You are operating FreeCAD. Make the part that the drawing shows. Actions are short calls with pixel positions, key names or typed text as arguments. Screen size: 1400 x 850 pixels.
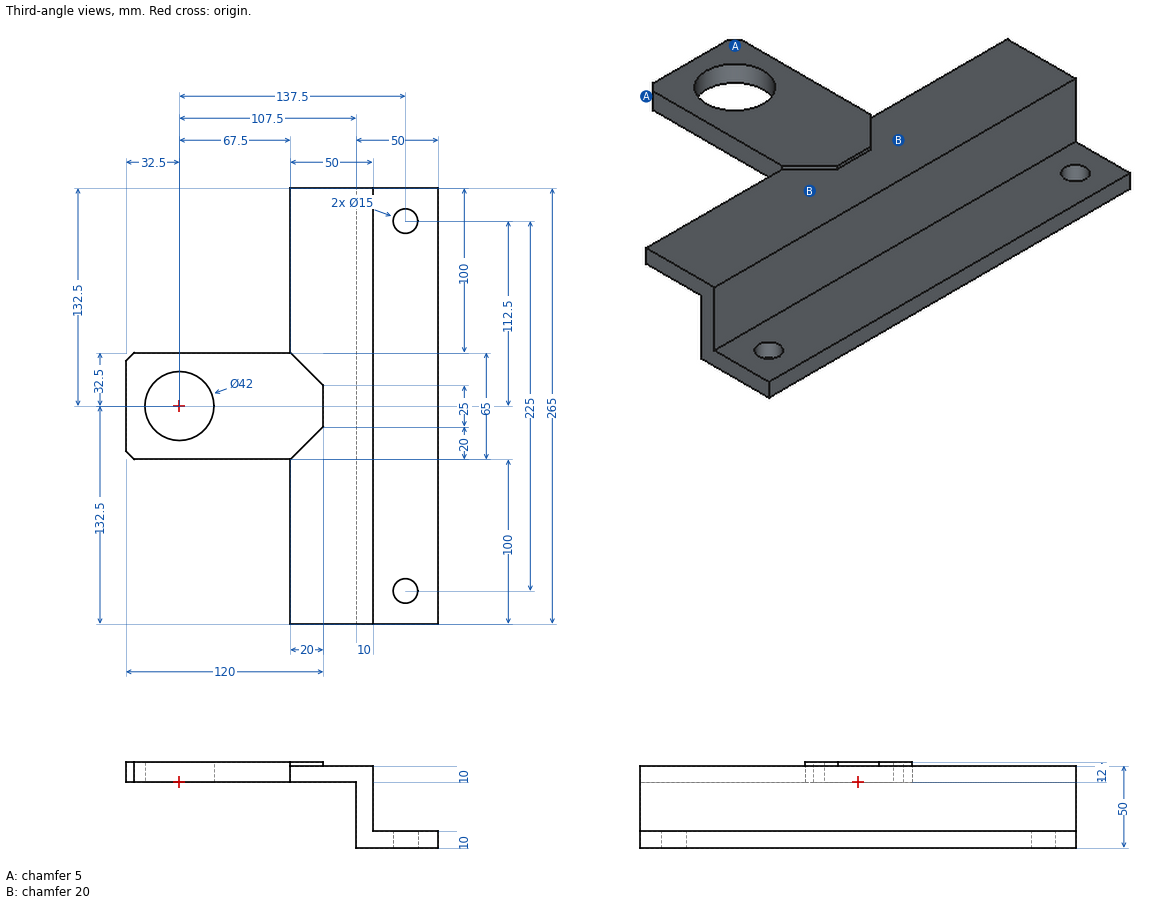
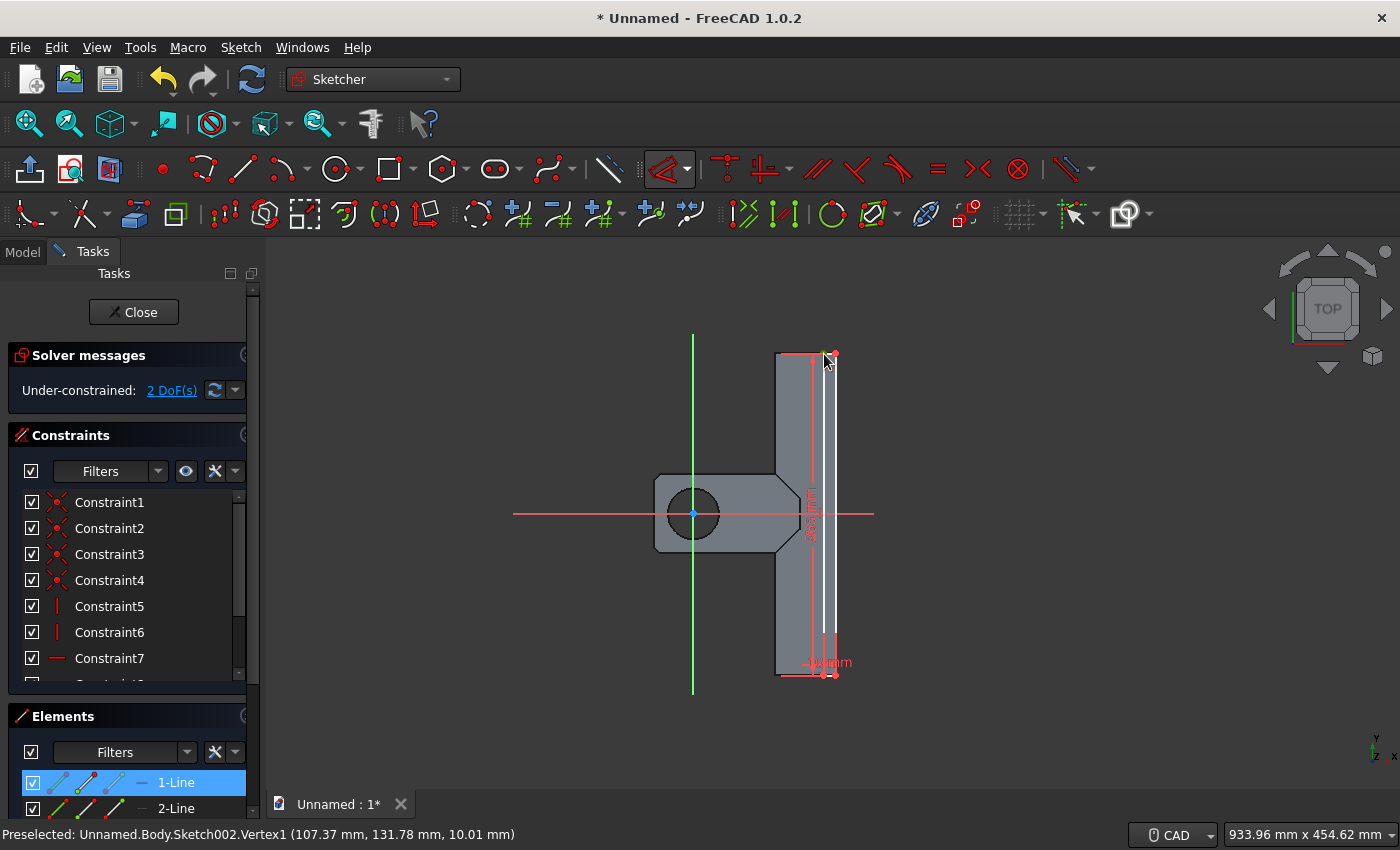
key(l)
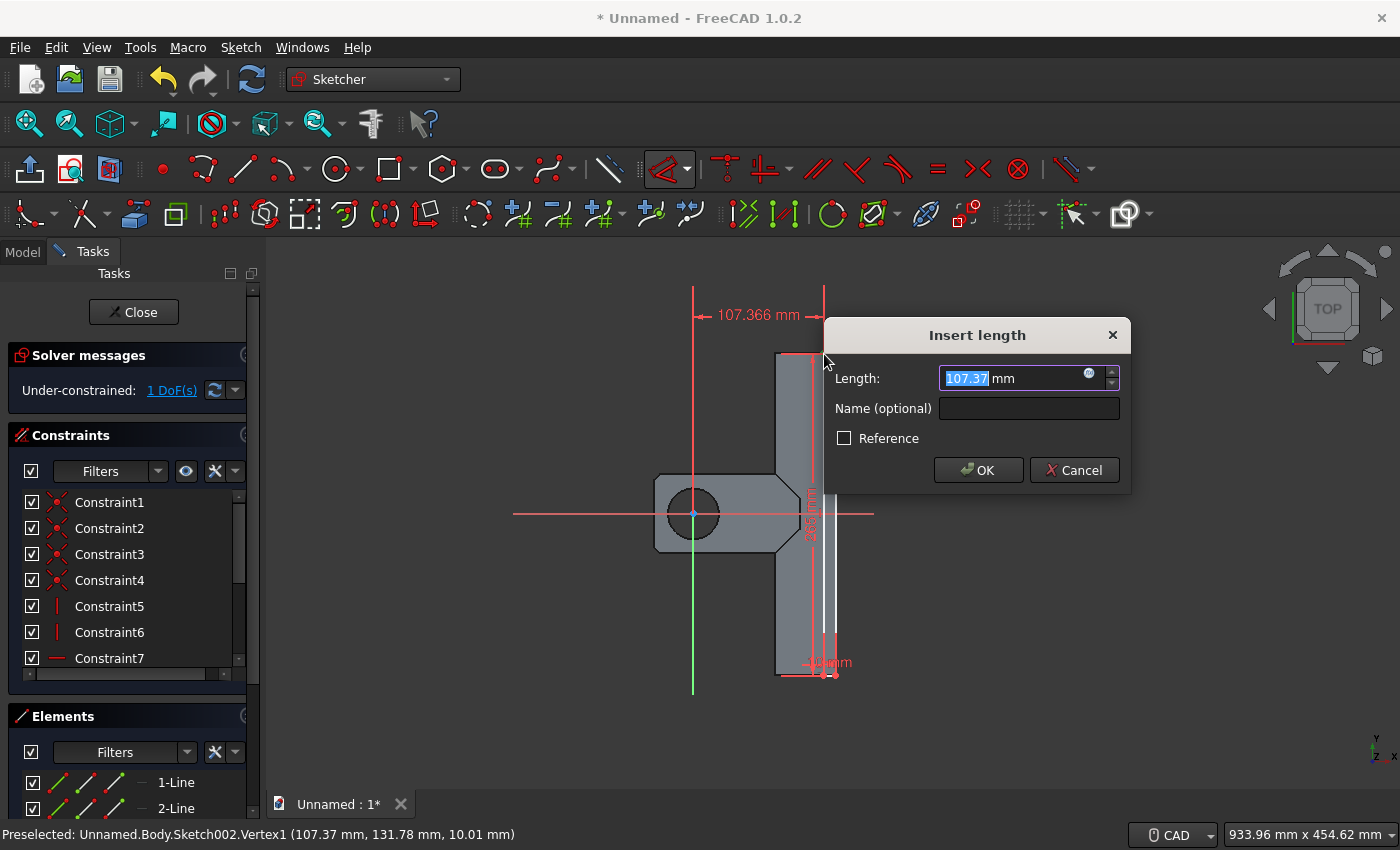
text(107.5)
key(Return)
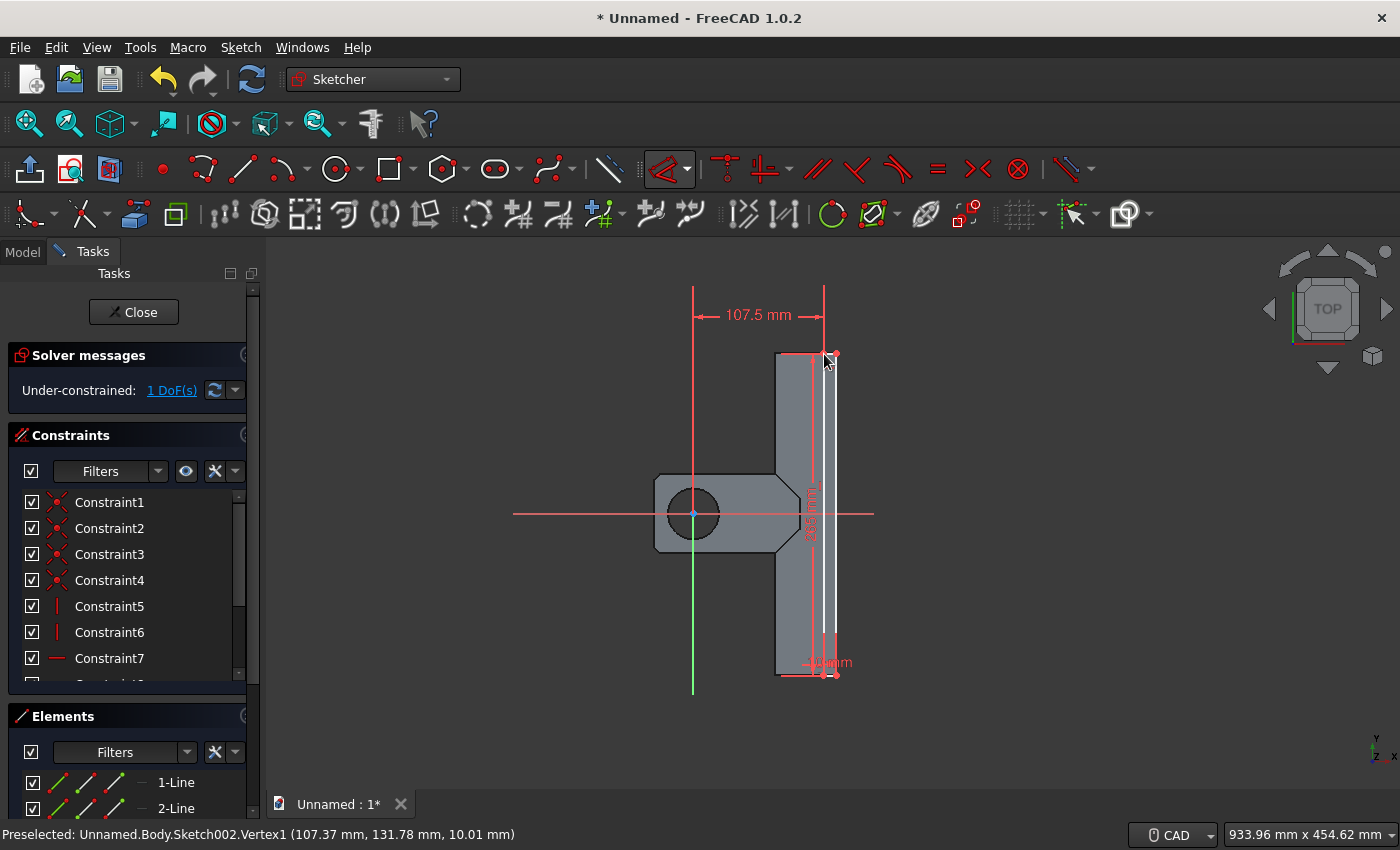
click(824, 354)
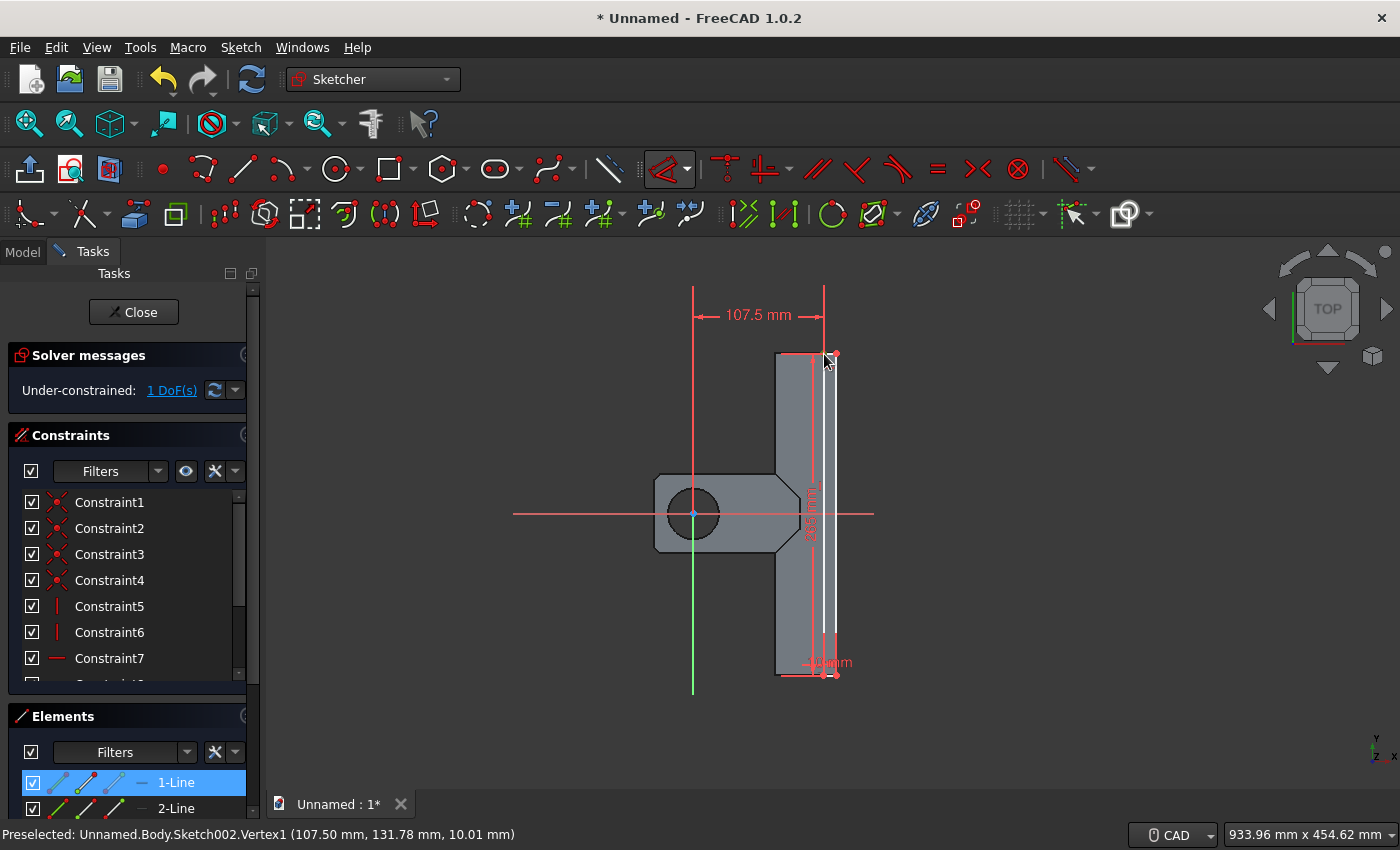
key(i)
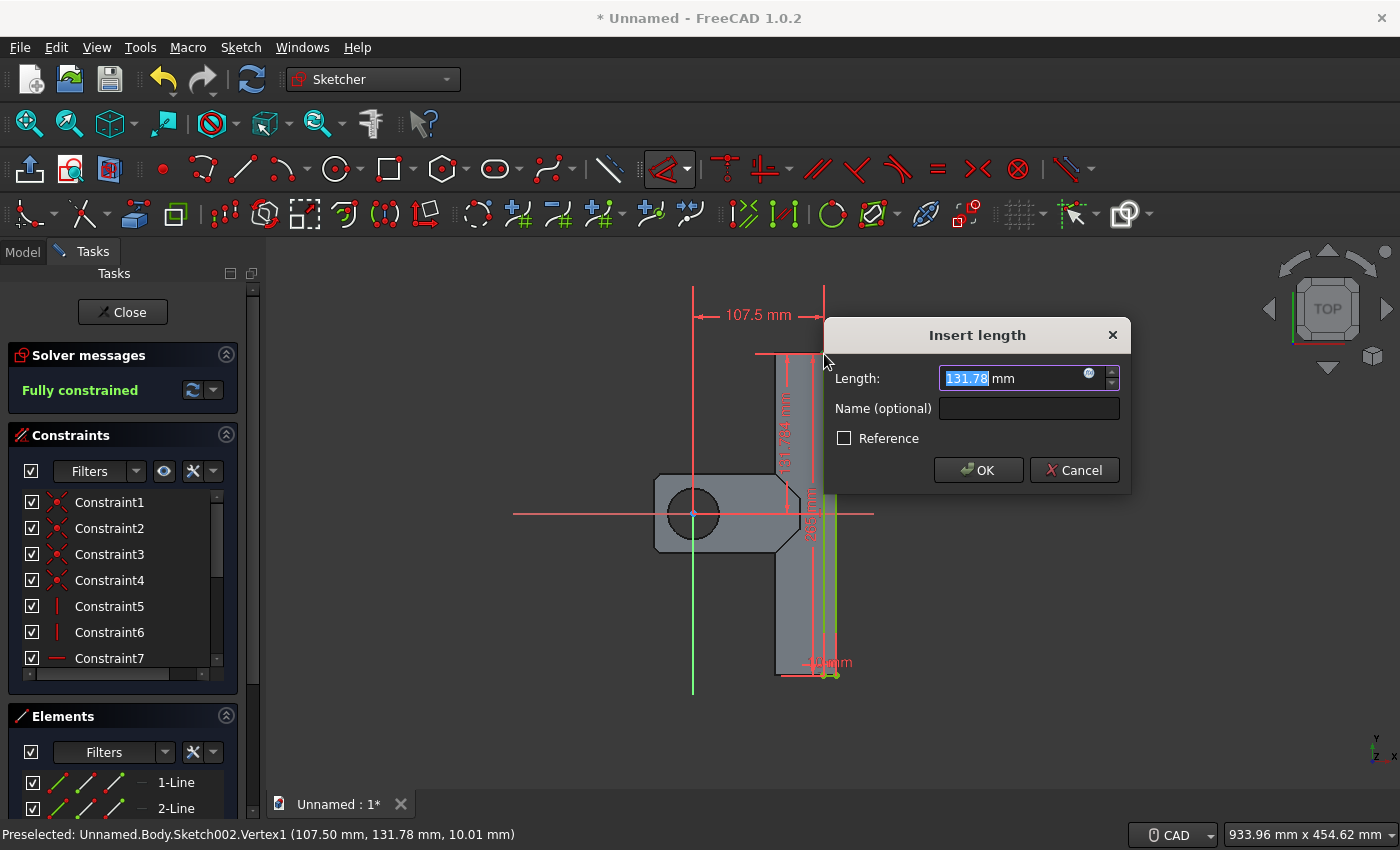
text(132.5)
key(Return)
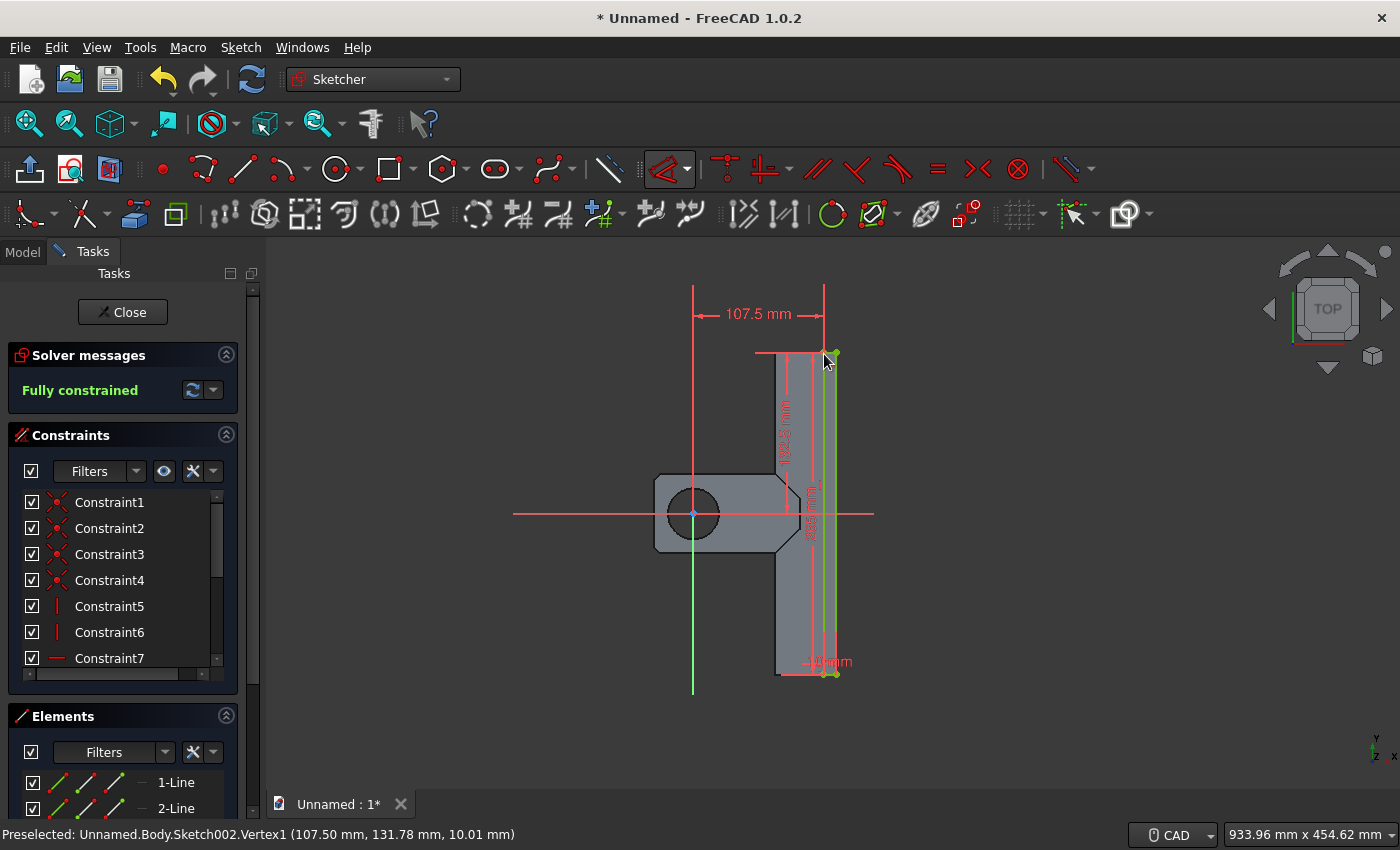
click(123, 312)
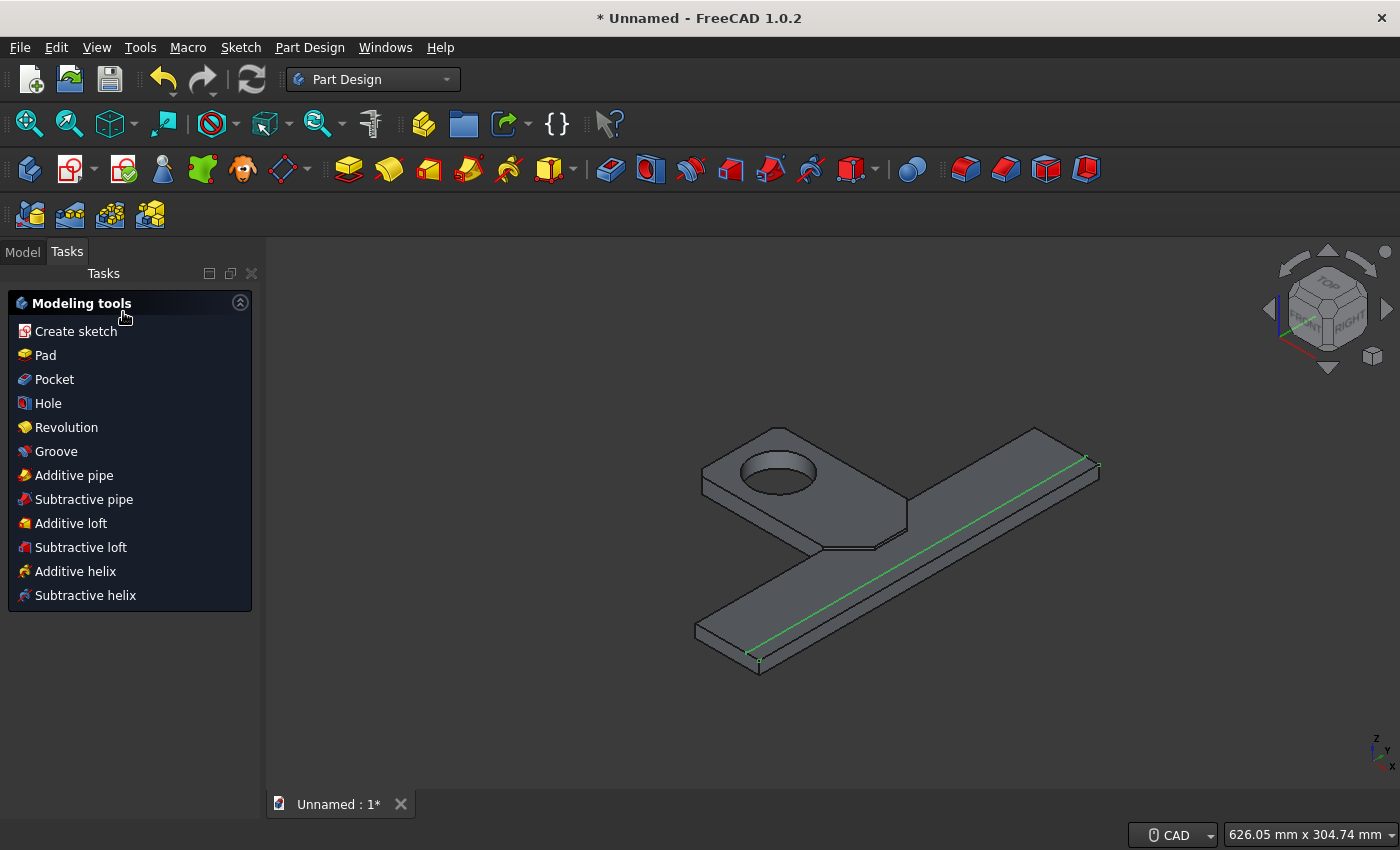
click(350, 170)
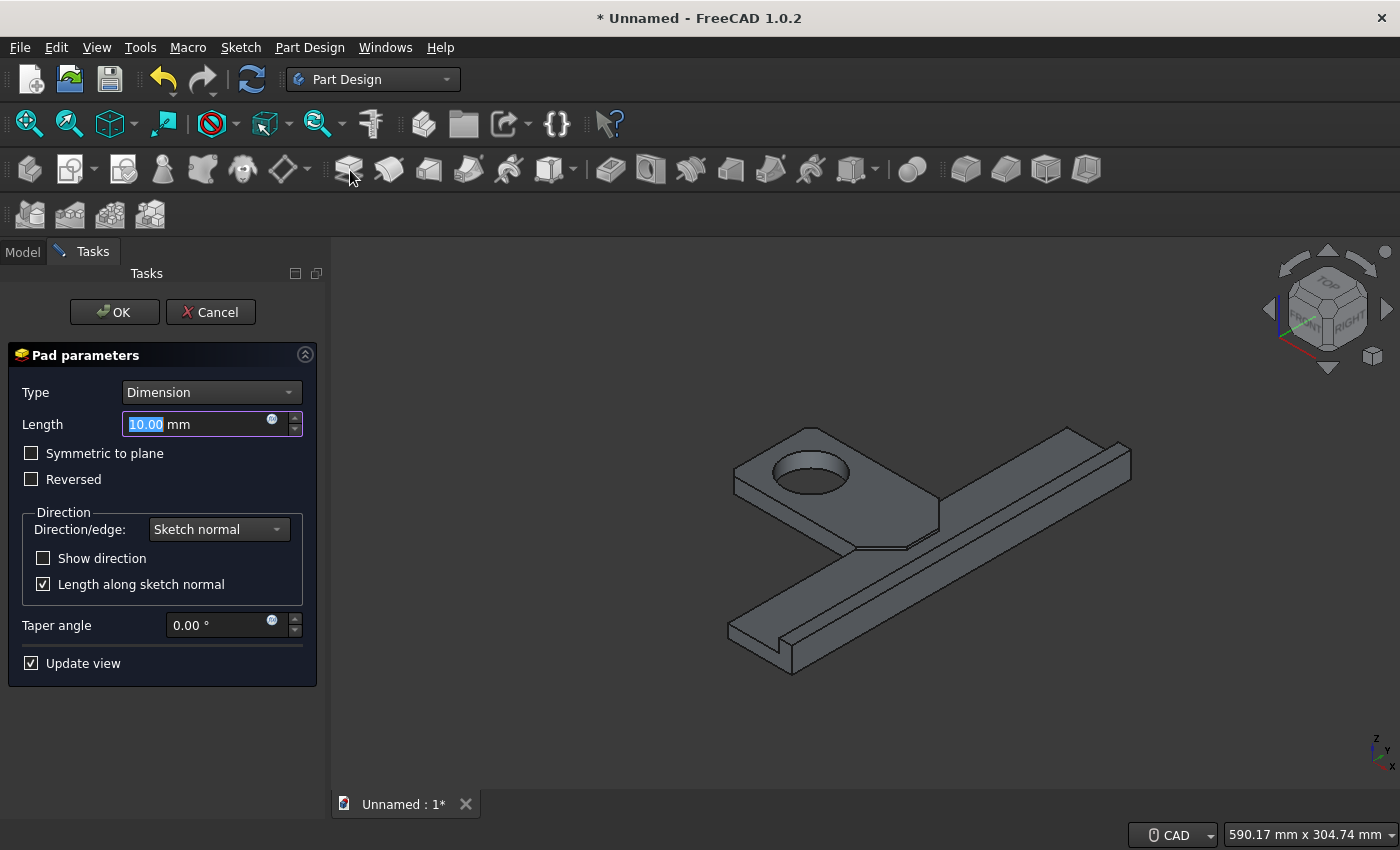
text(50)
key(Tab)